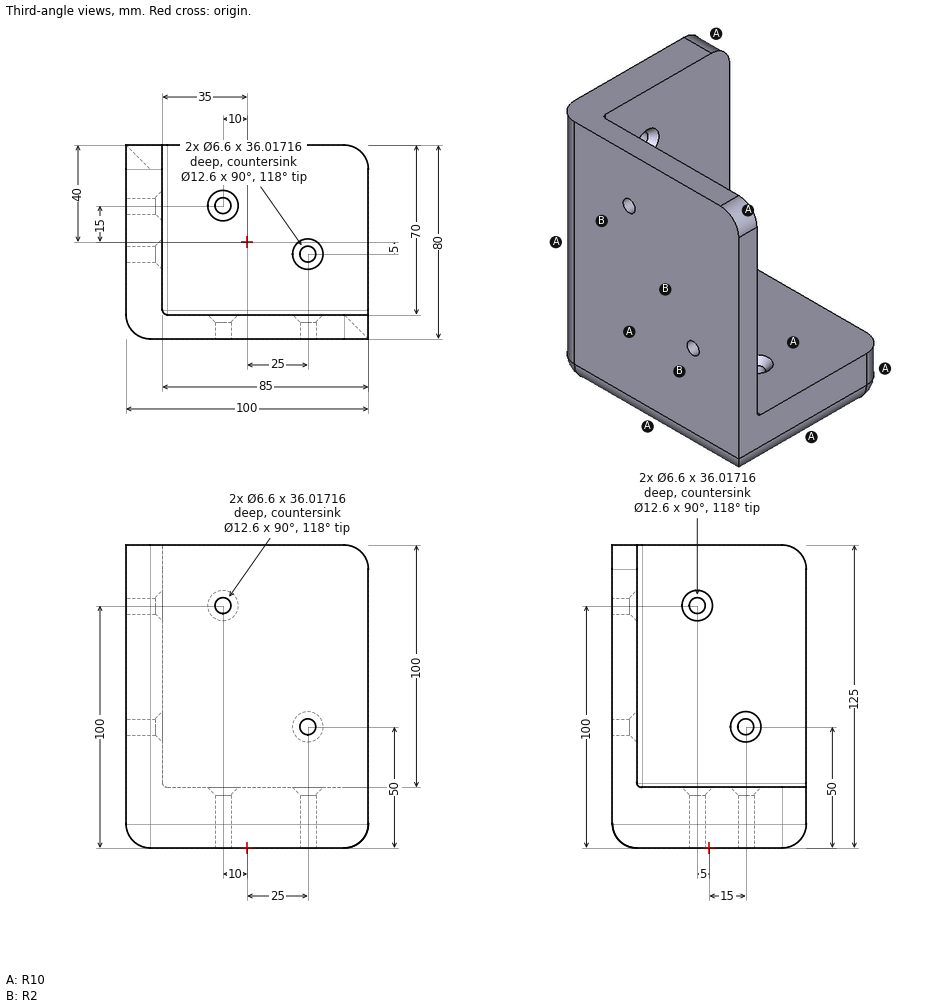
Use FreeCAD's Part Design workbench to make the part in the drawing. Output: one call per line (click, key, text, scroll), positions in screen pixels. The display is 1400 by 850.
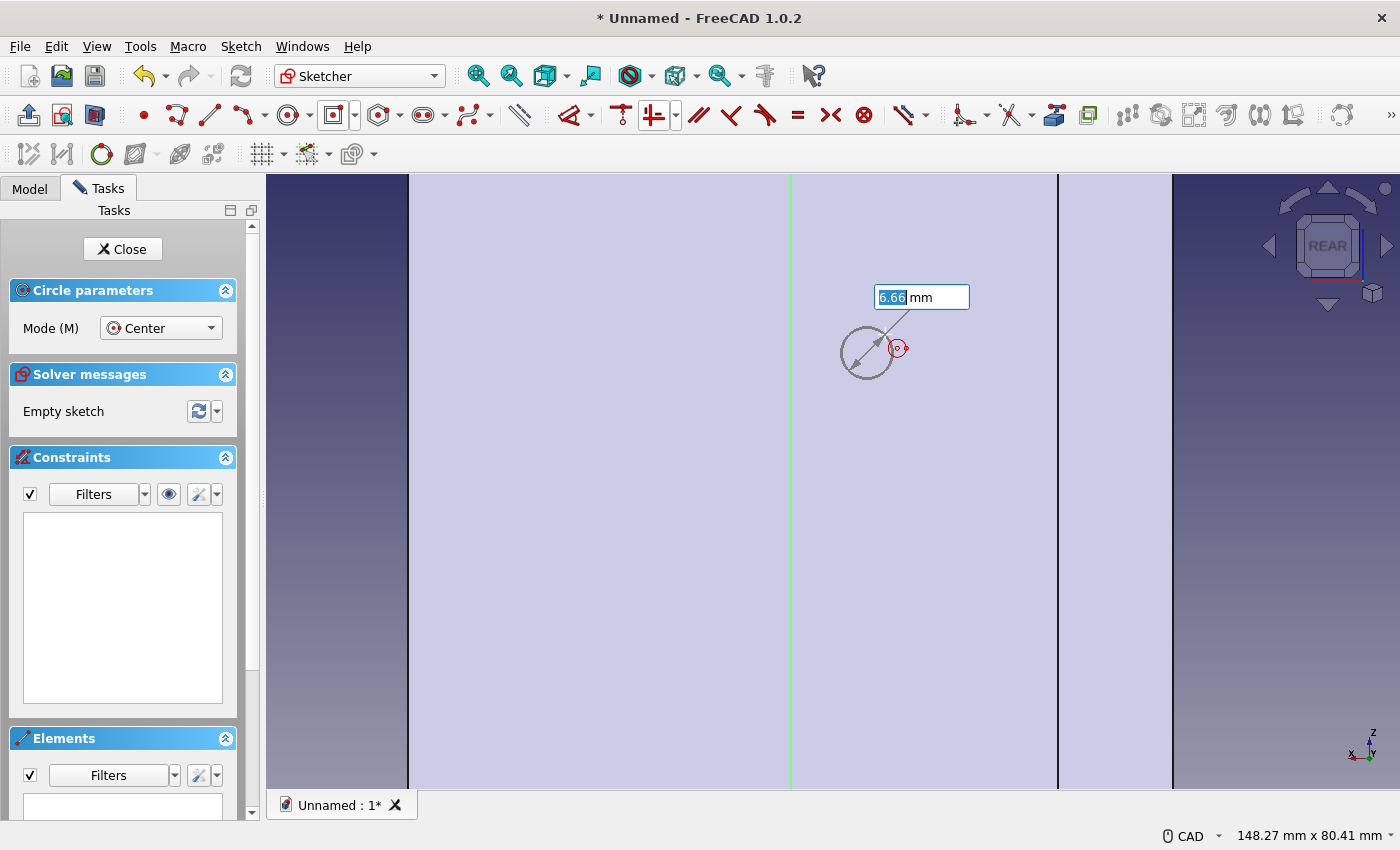
text(6.6)
key(Return)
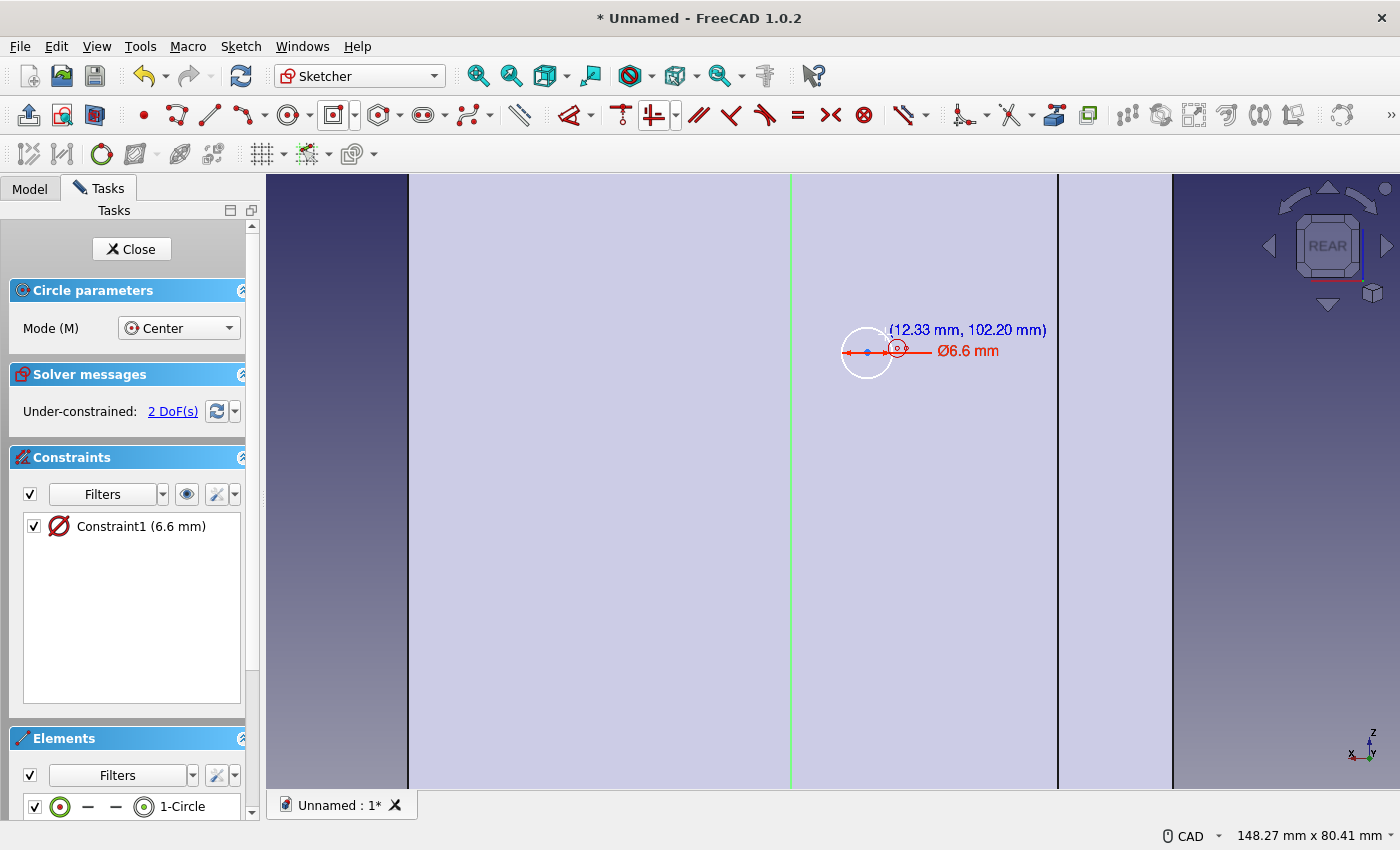
click(599, 734)
move(617, 716)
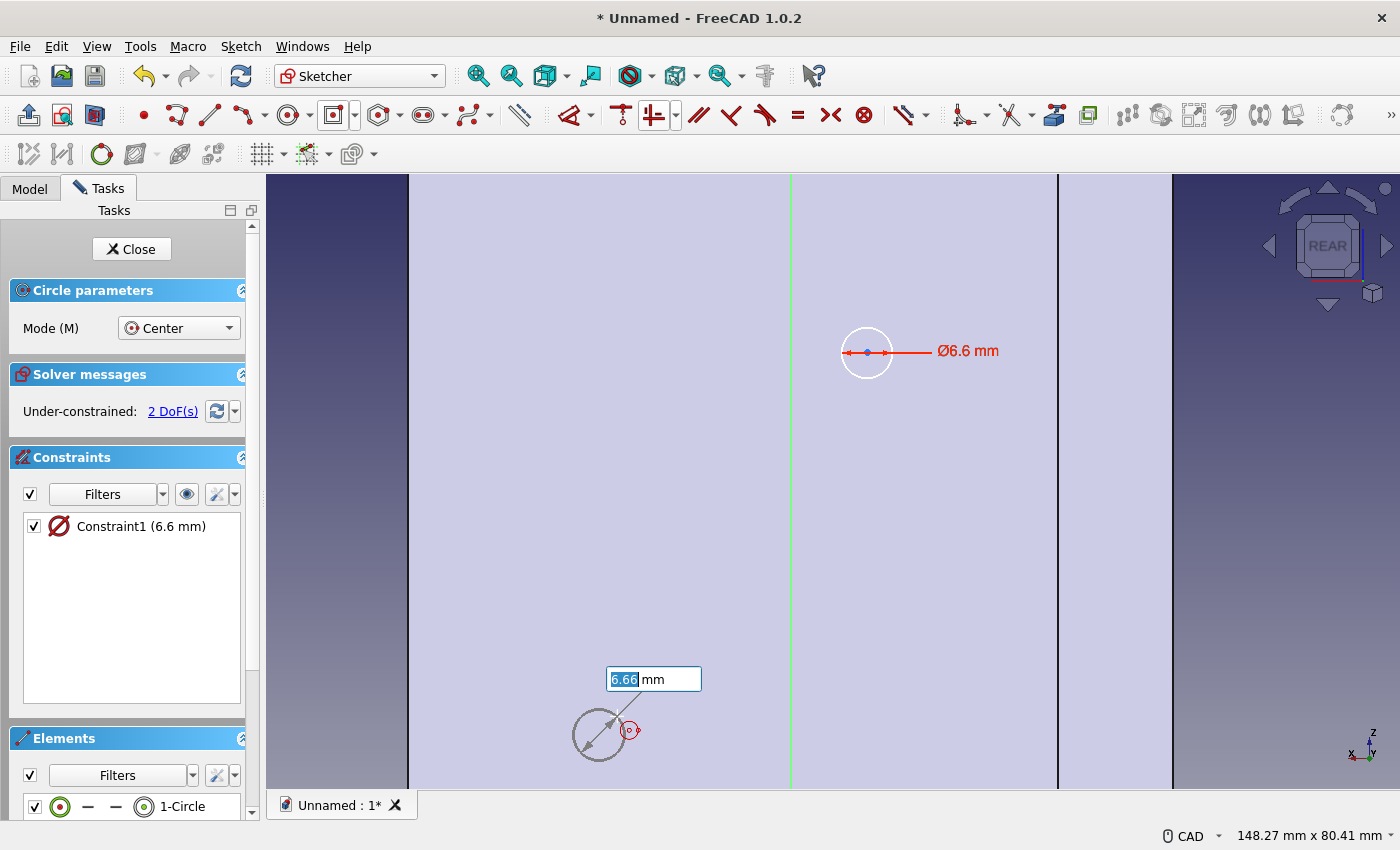
text(6.6)
key(Return)
key(Escape)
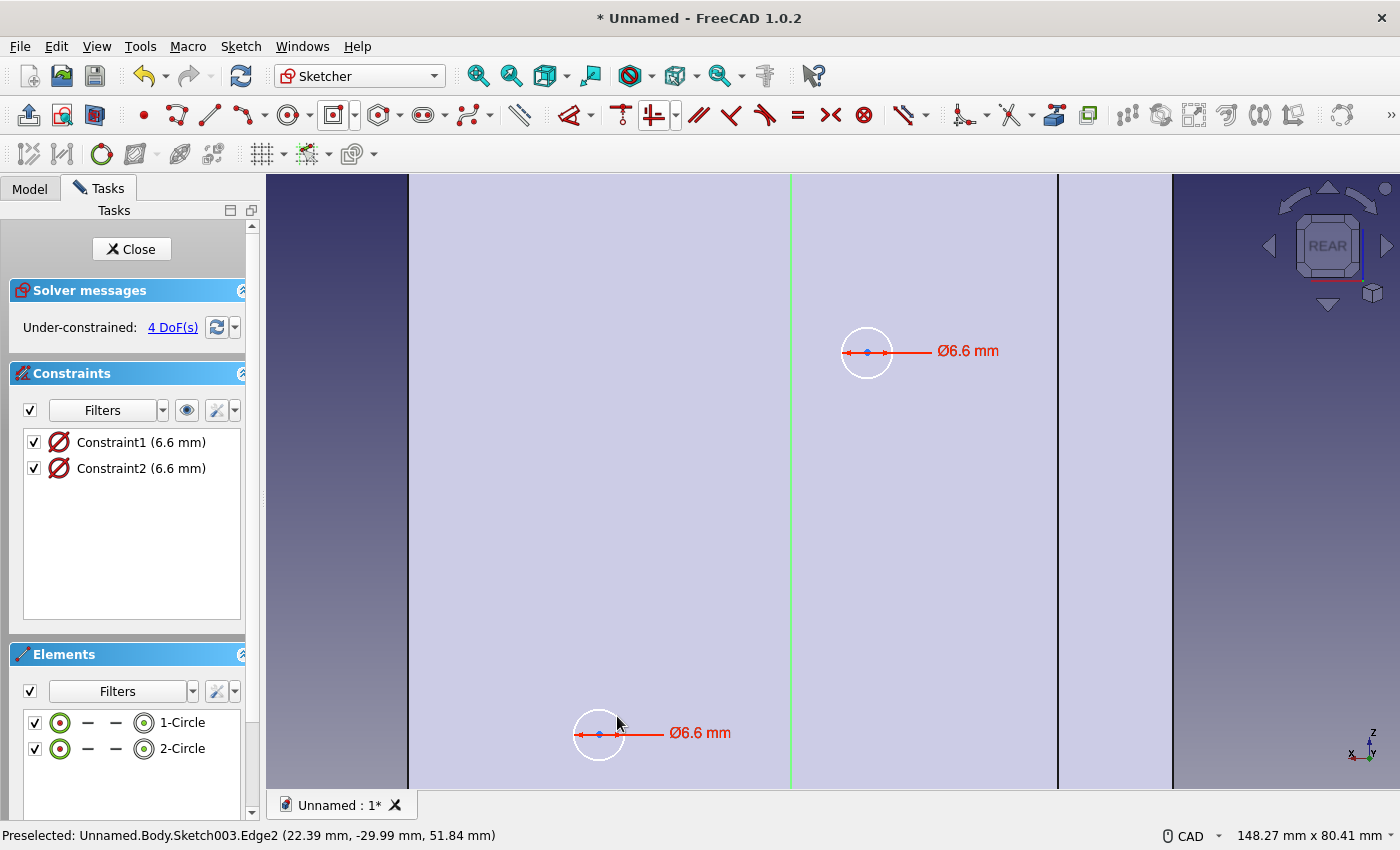
key(d)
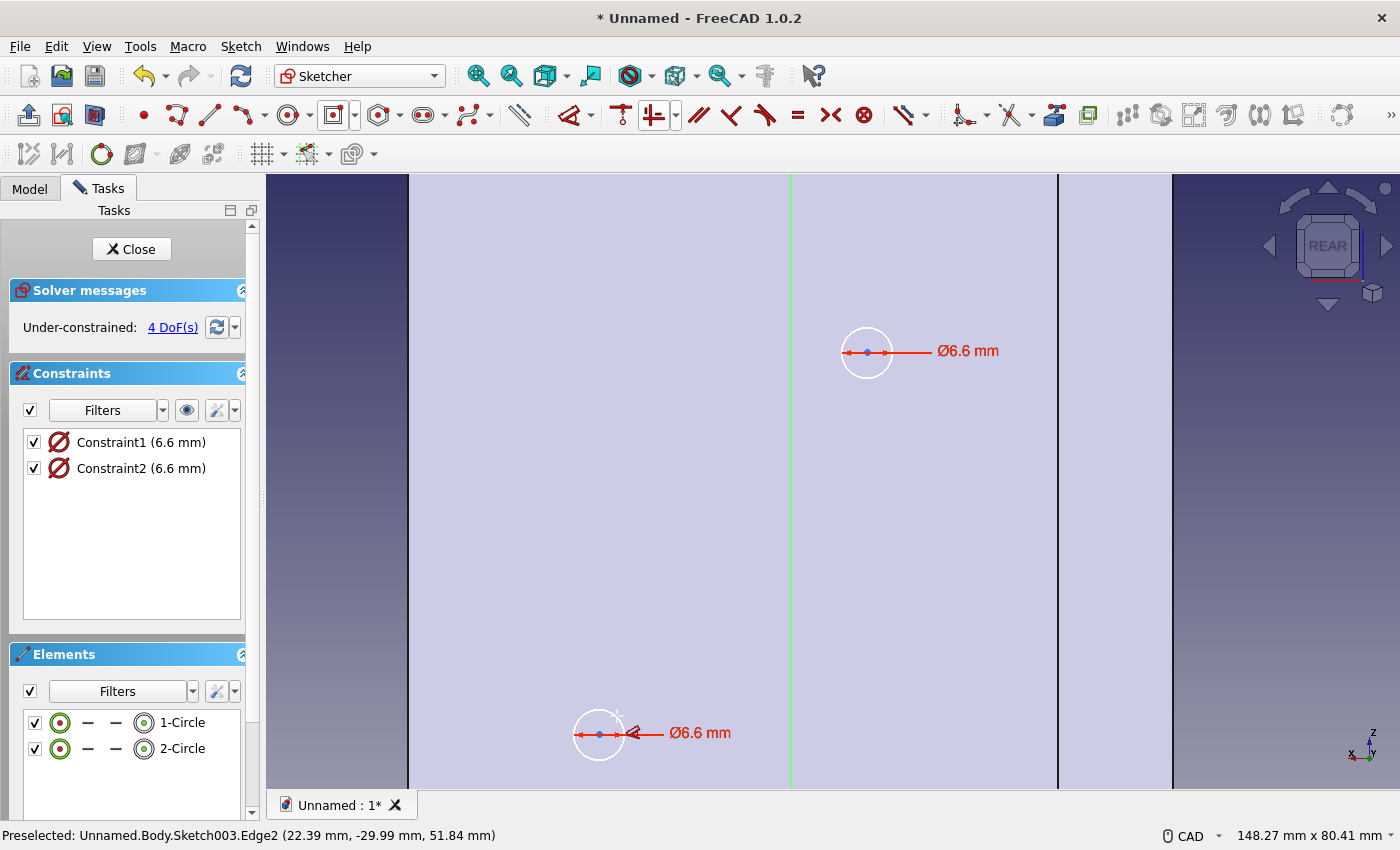
click(867, 353)
click(829, 319)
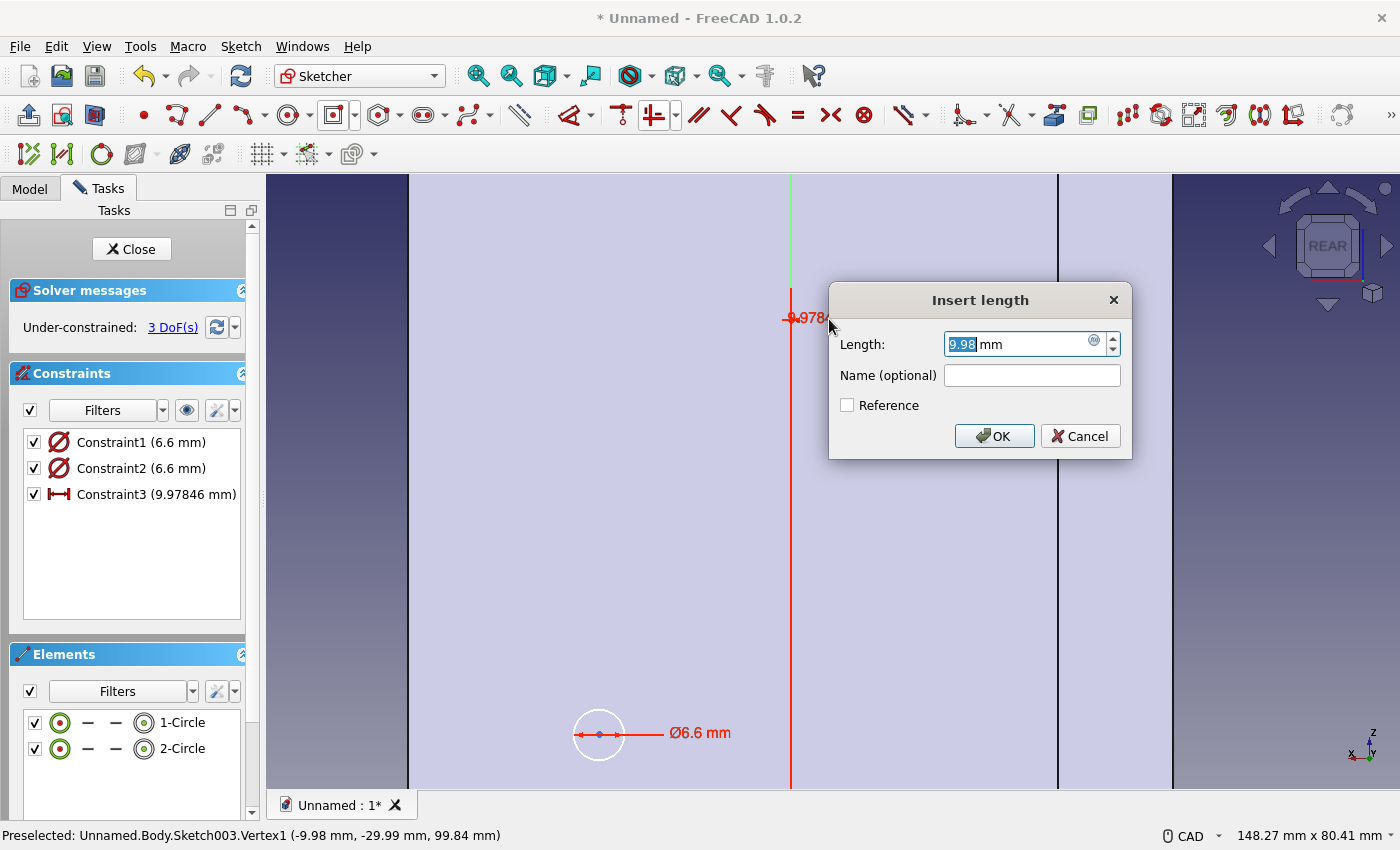
text(10)
key(Return)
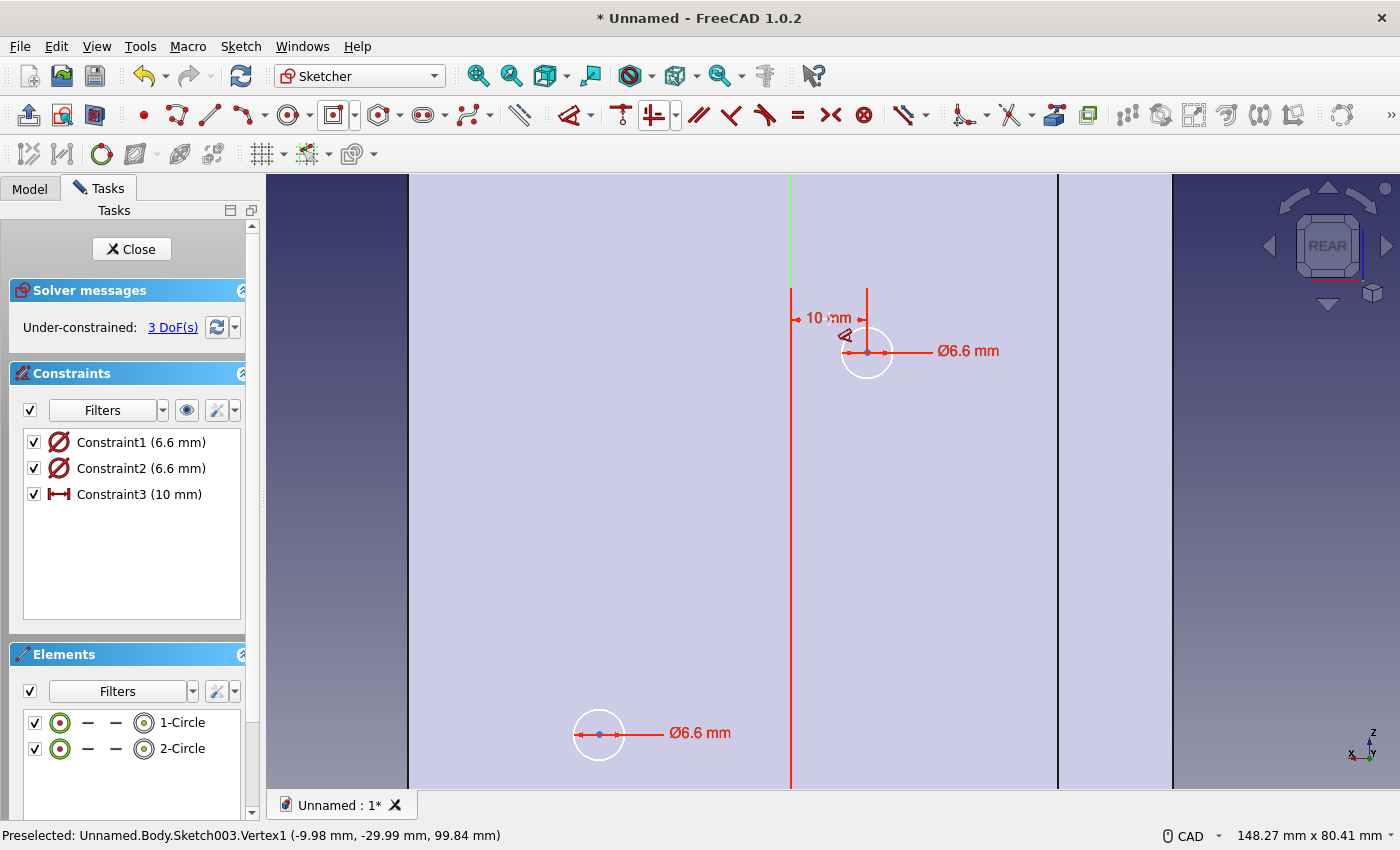
click(599, 735)
click(695, 701)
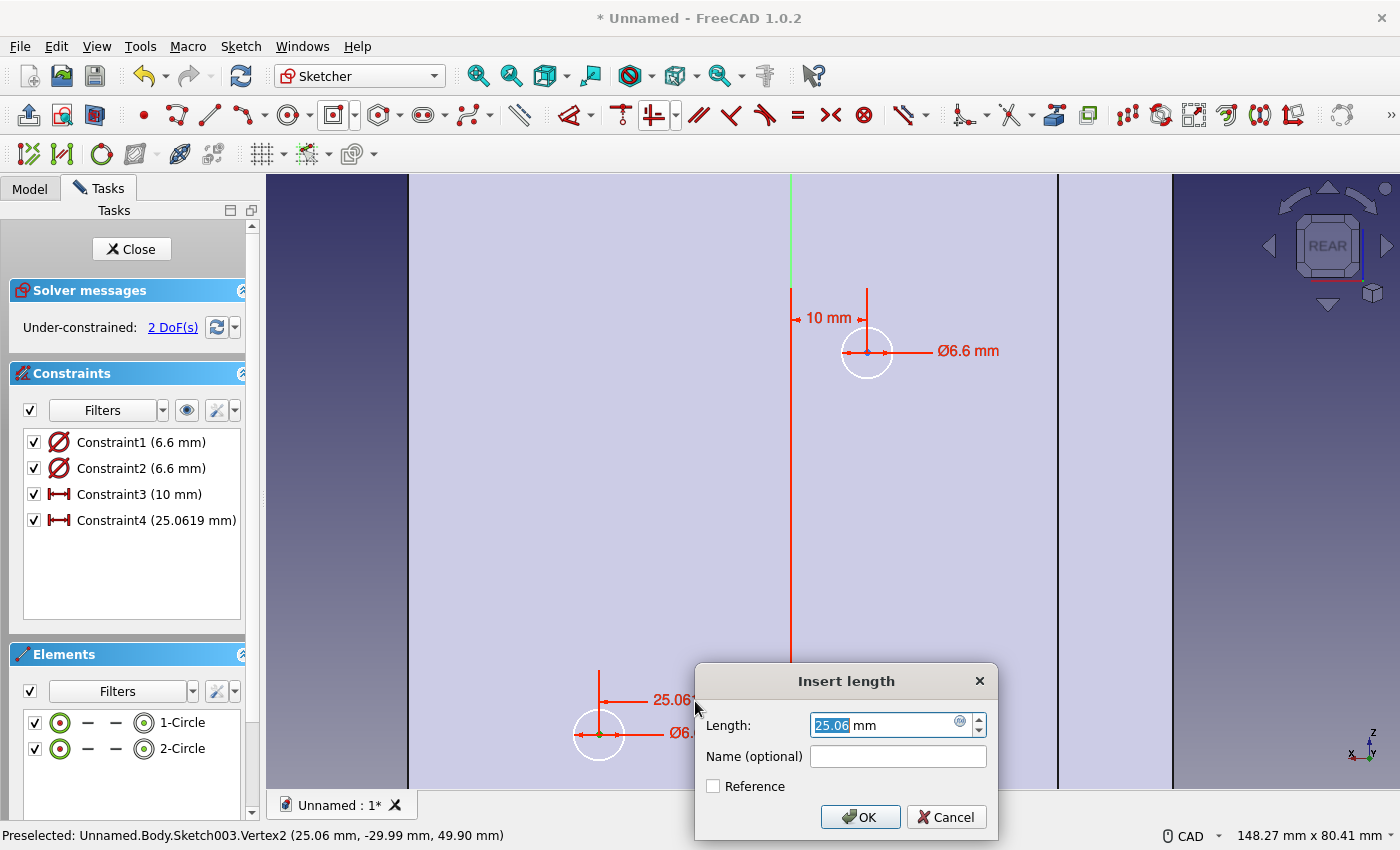
text(25)
key(Return)